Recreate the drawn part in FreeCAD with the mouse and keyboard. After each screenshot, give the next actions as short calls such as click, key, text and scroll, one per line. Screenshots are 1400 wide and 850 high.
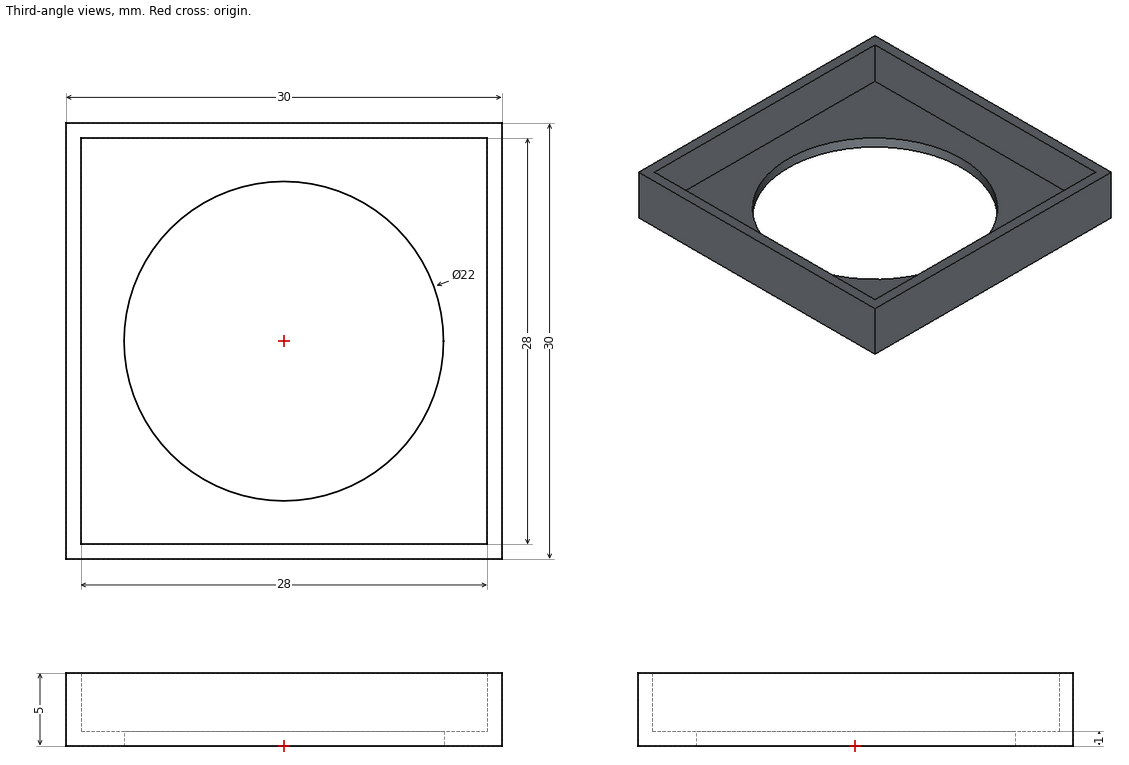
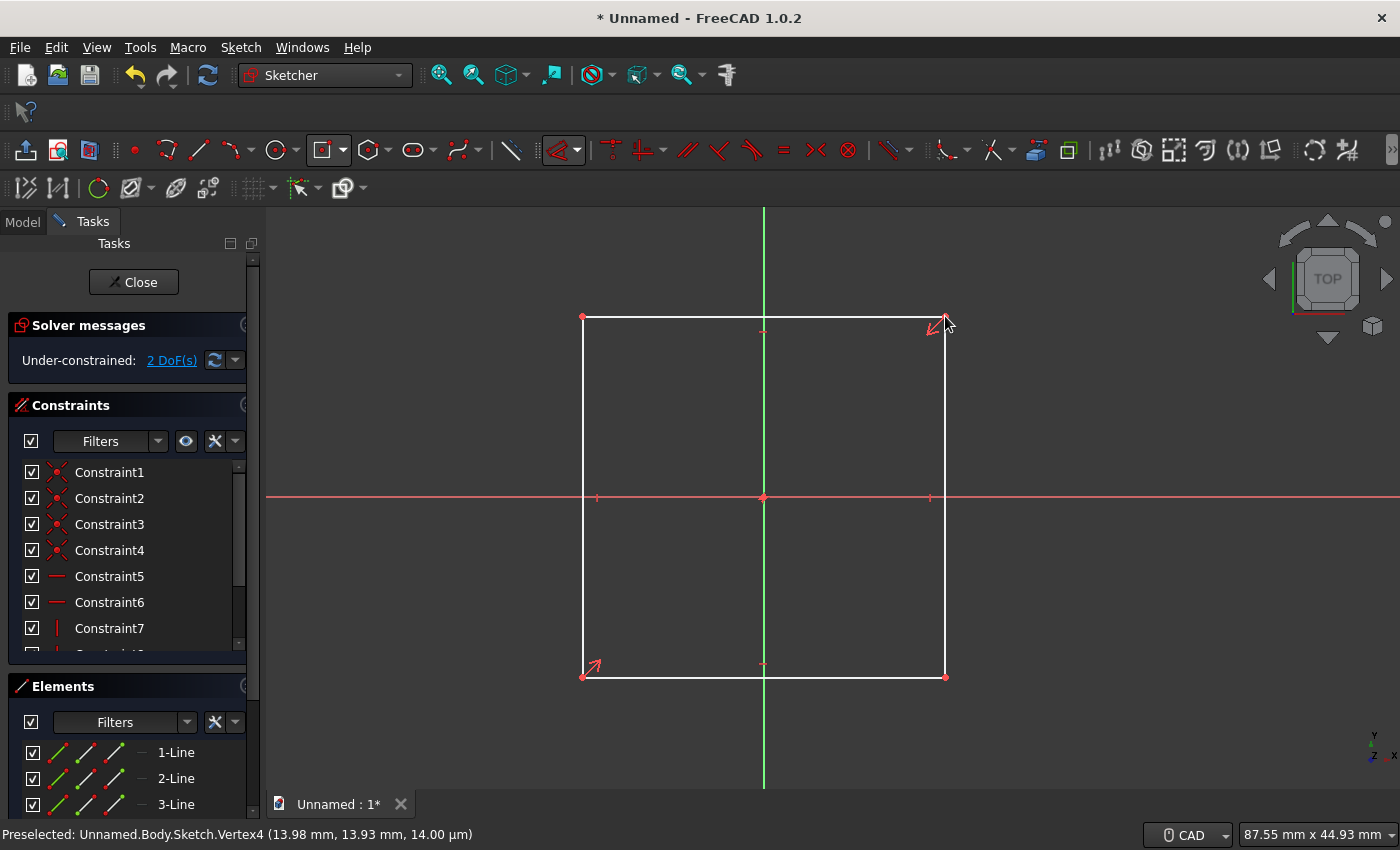
click(558, 150)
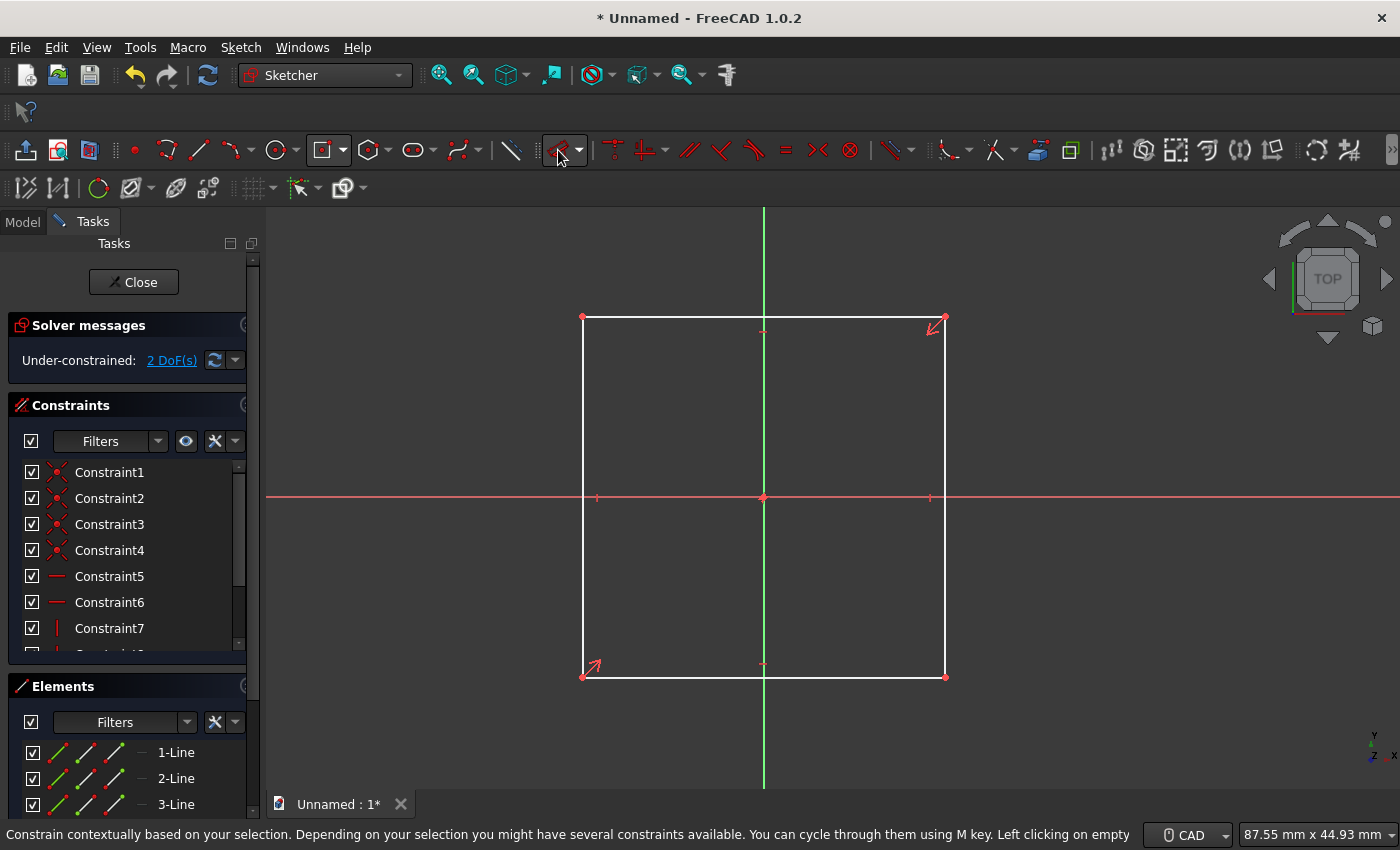
click(692, 678)
click(681, 712)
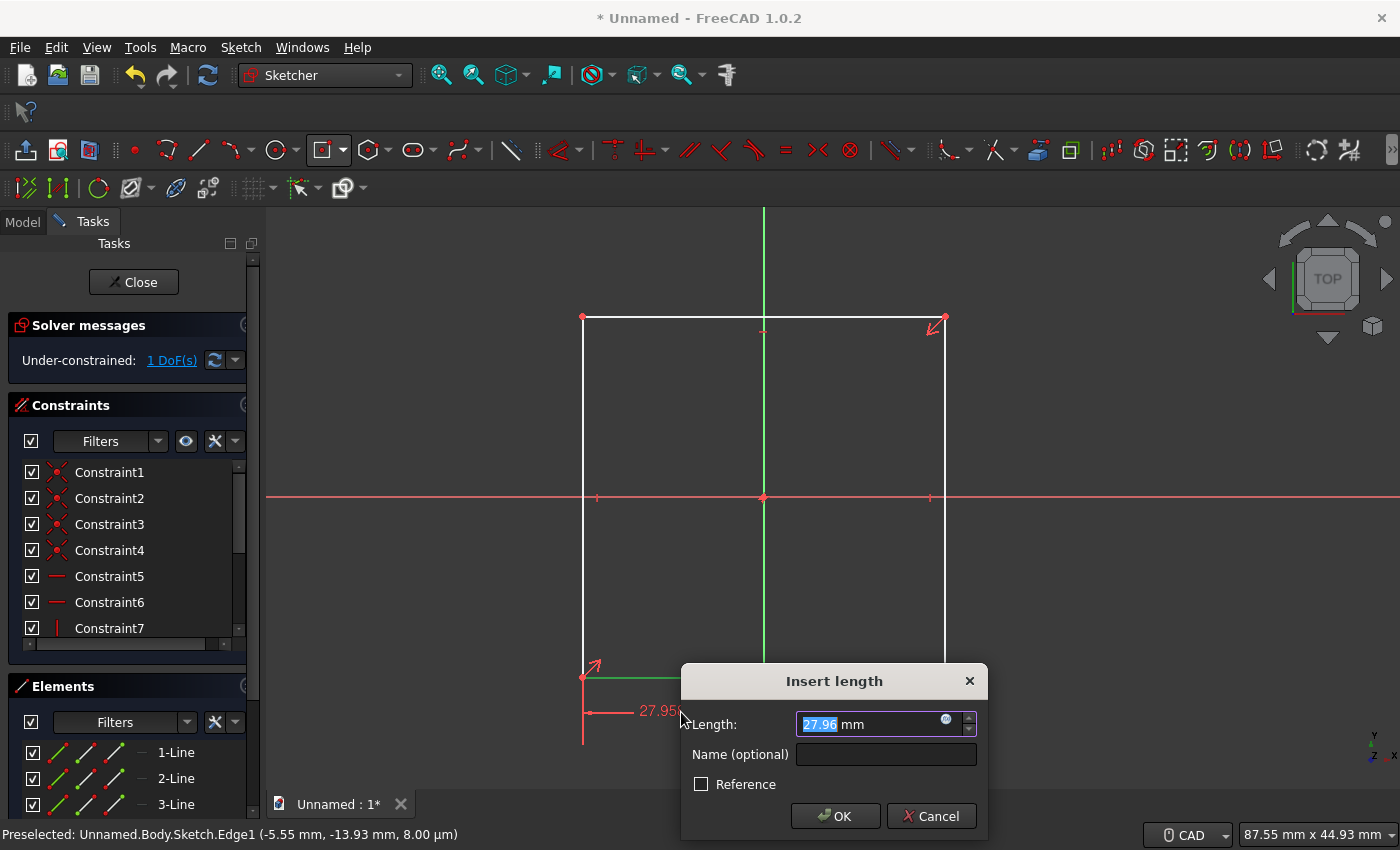
text(28)
key(Return)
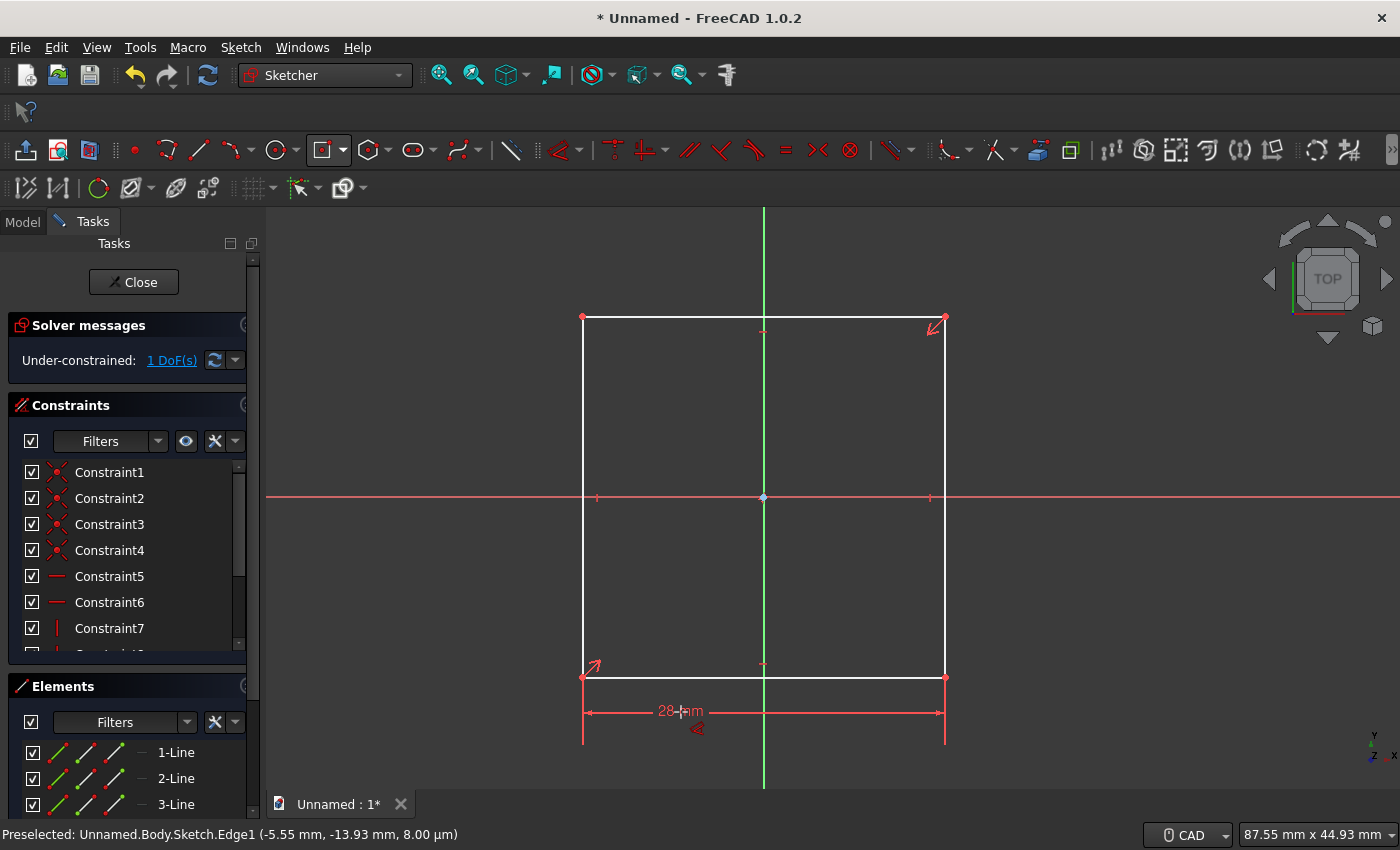
click(945, 570)
click(979, 414)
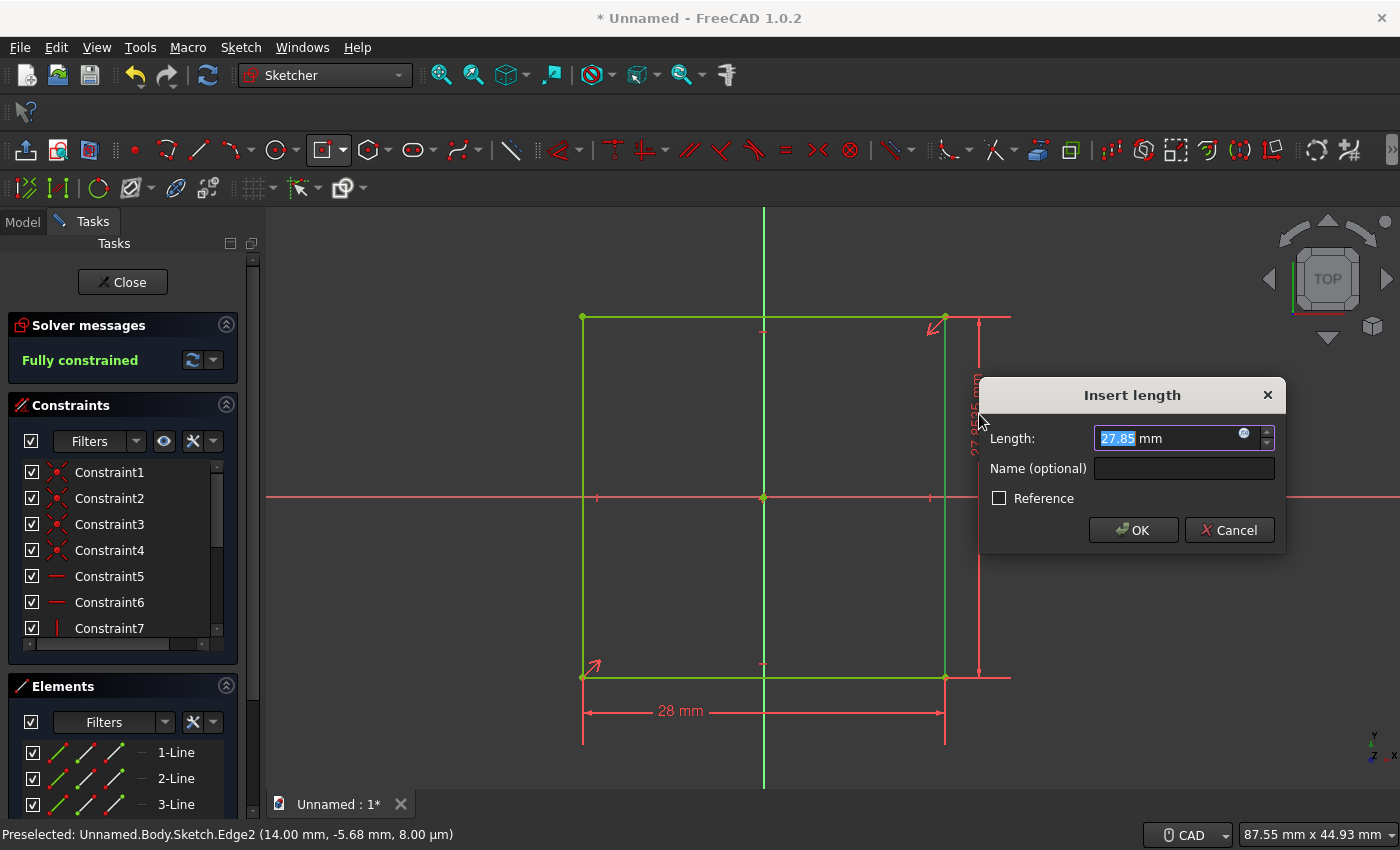
text(28)
key(Return)
key(Escape)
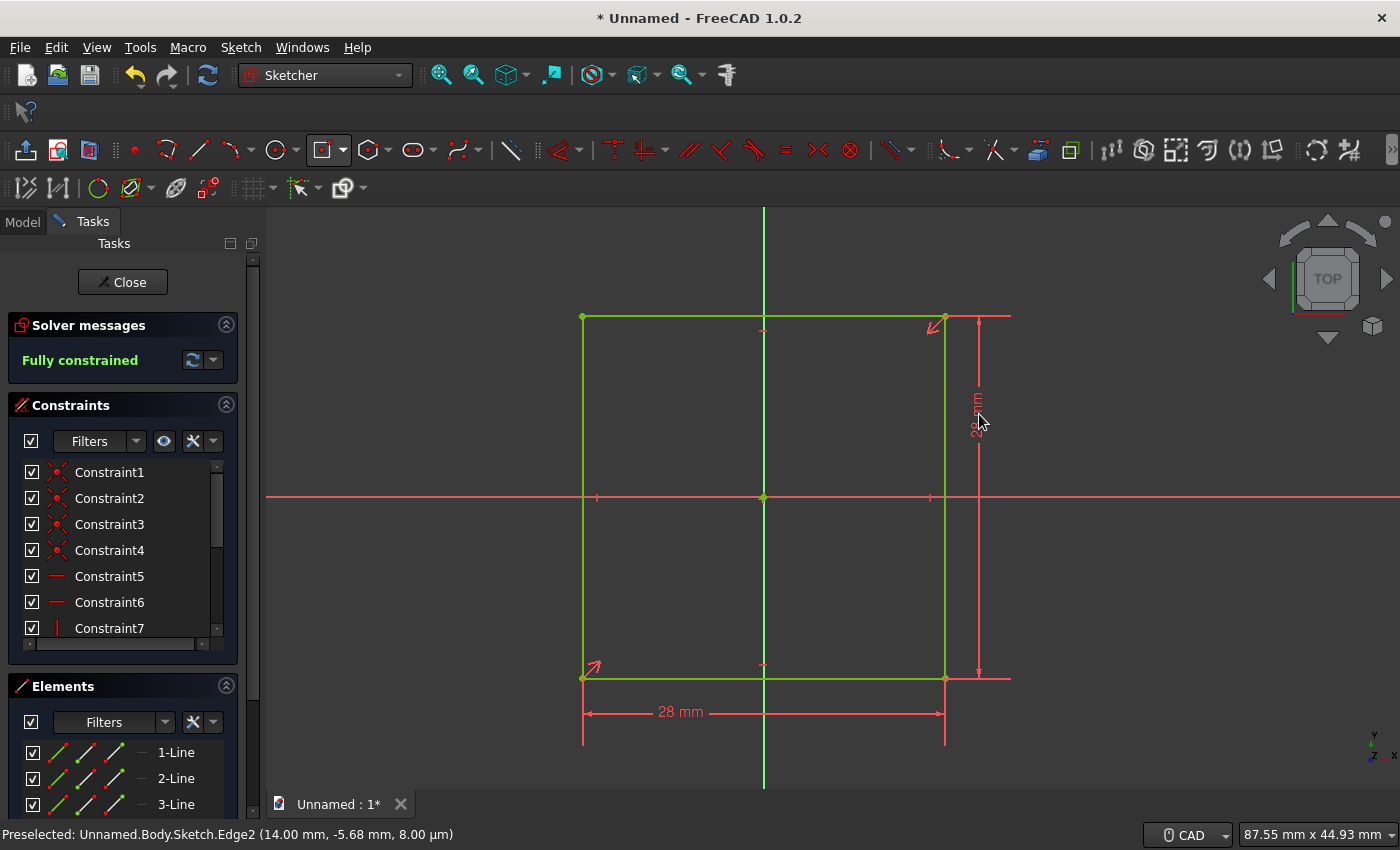
click(123, 282)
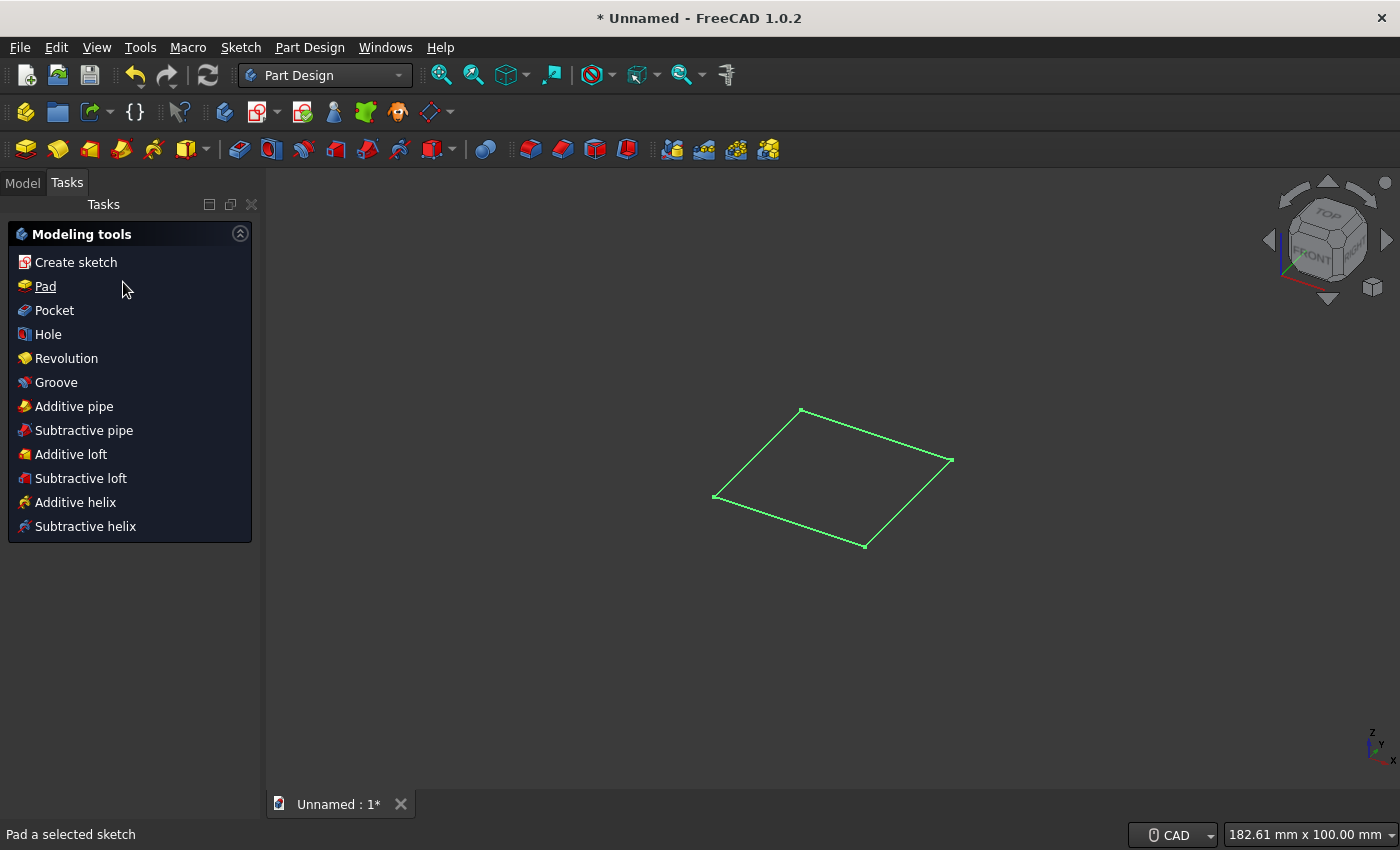
click(26, 150)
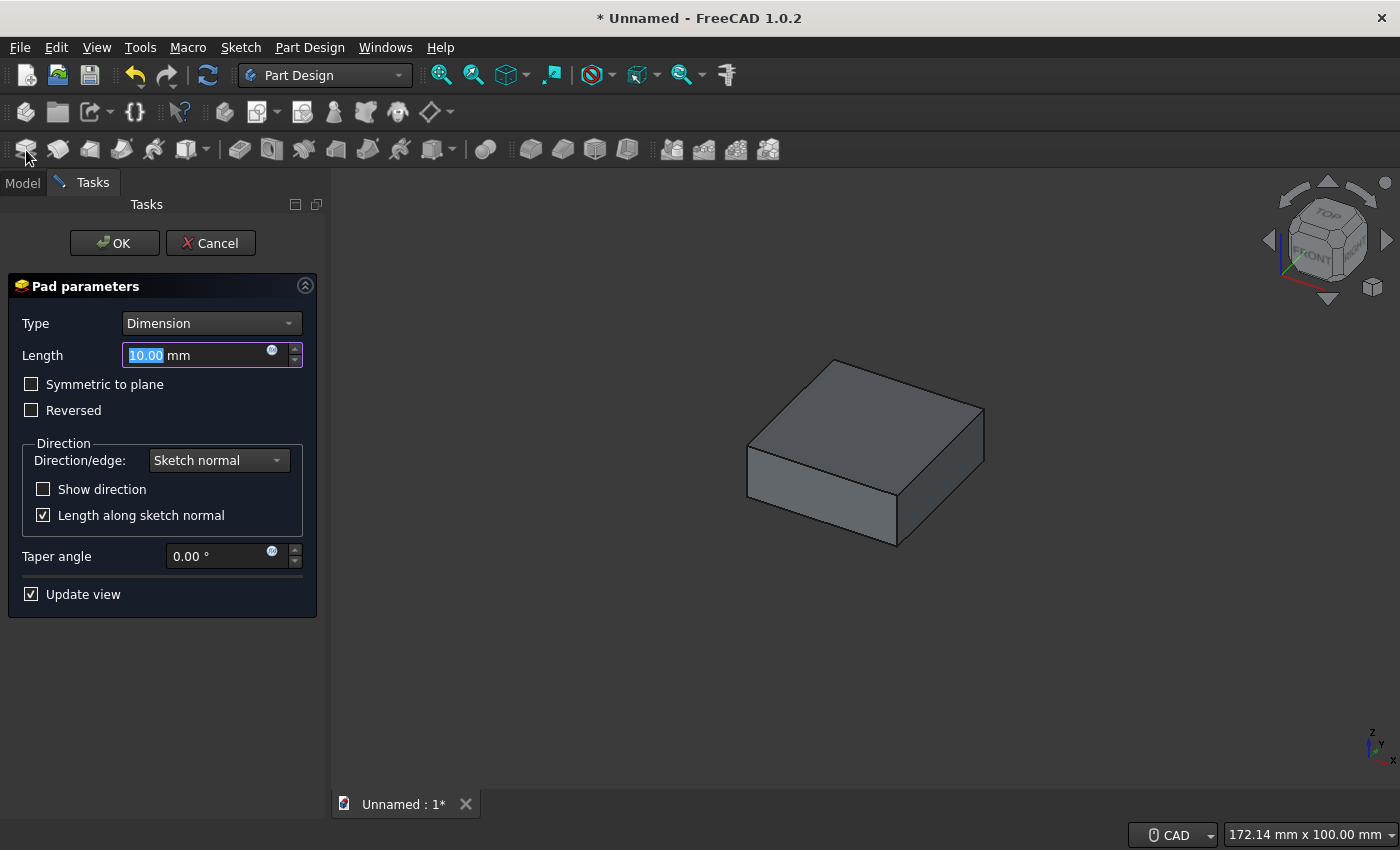
text(1)
key(Tab)